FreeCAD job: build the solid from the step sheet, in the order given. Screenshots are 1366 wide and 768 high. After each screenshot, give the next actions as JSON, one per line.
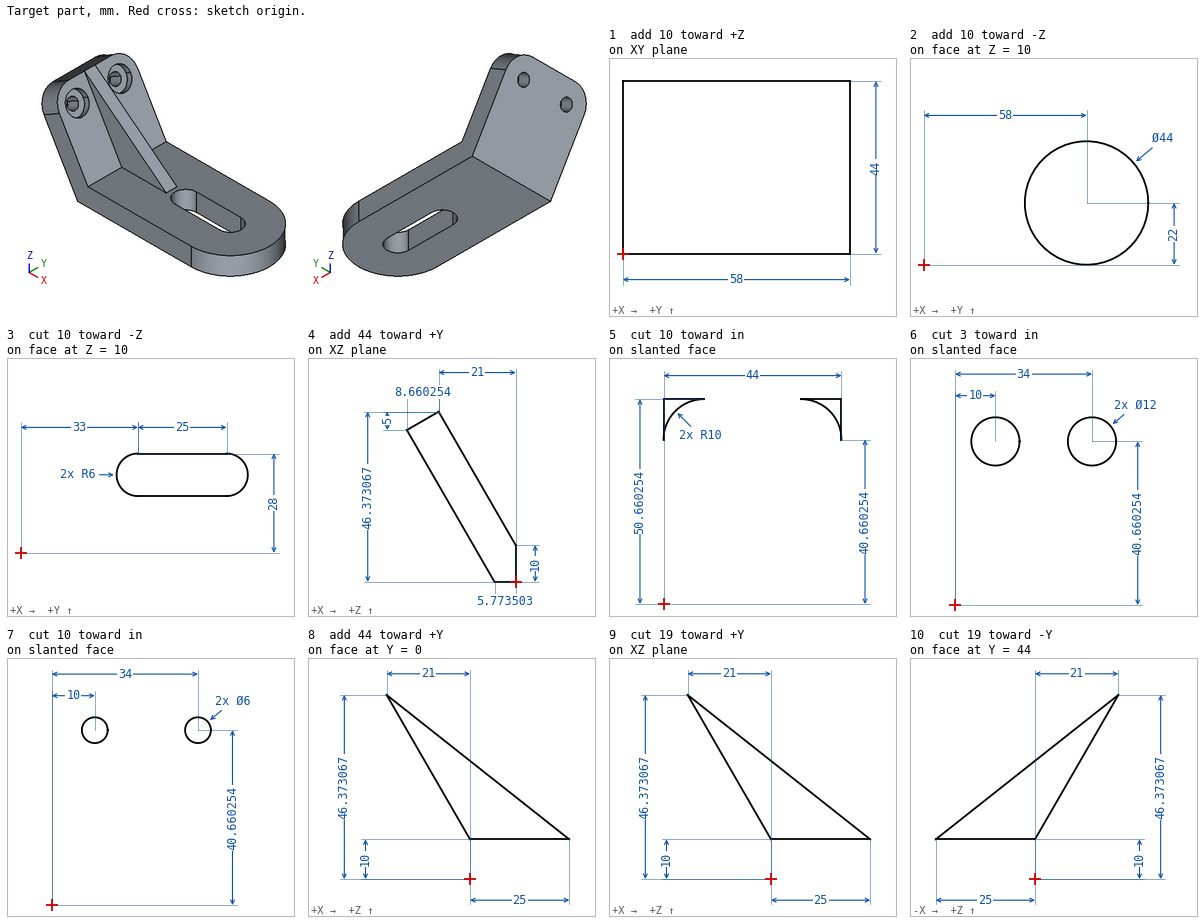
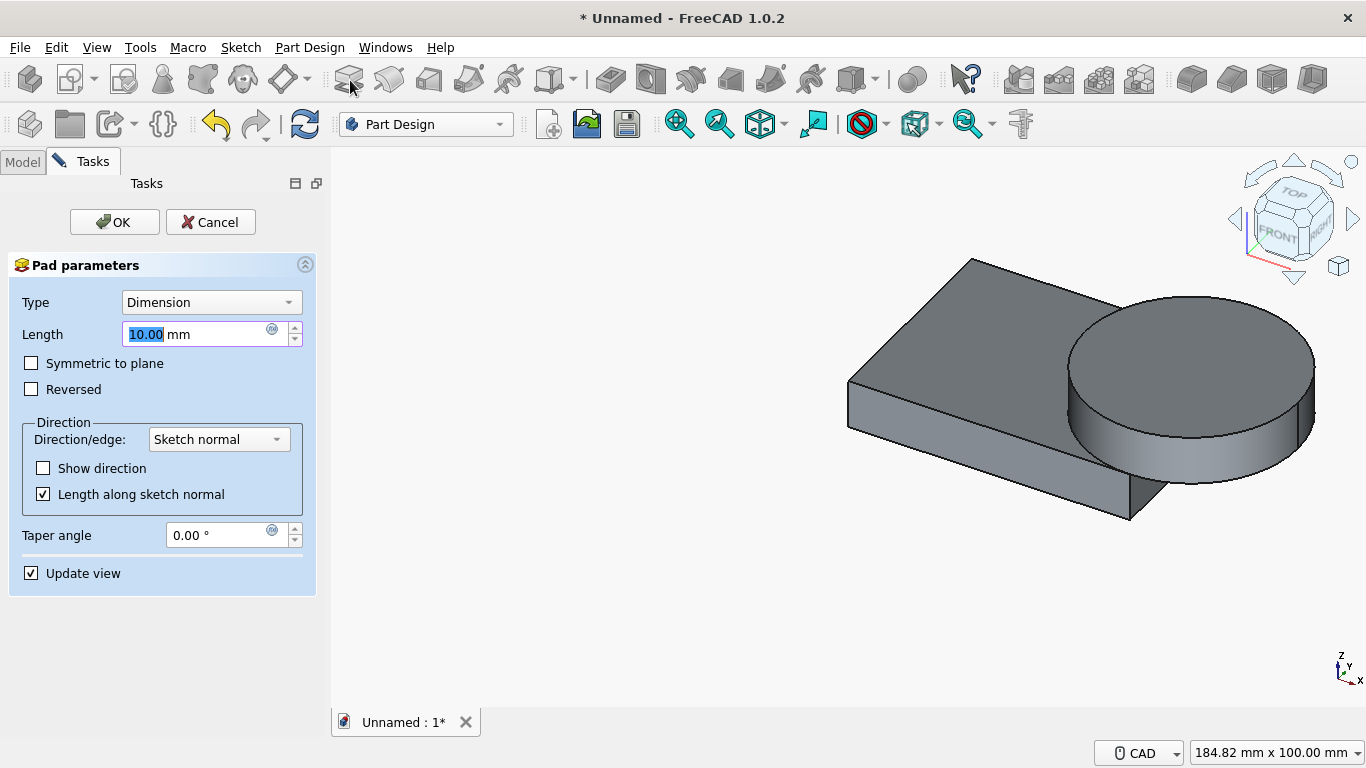
{"action": "type", "text": "10"}
{"action": "key", "text": "Tab"}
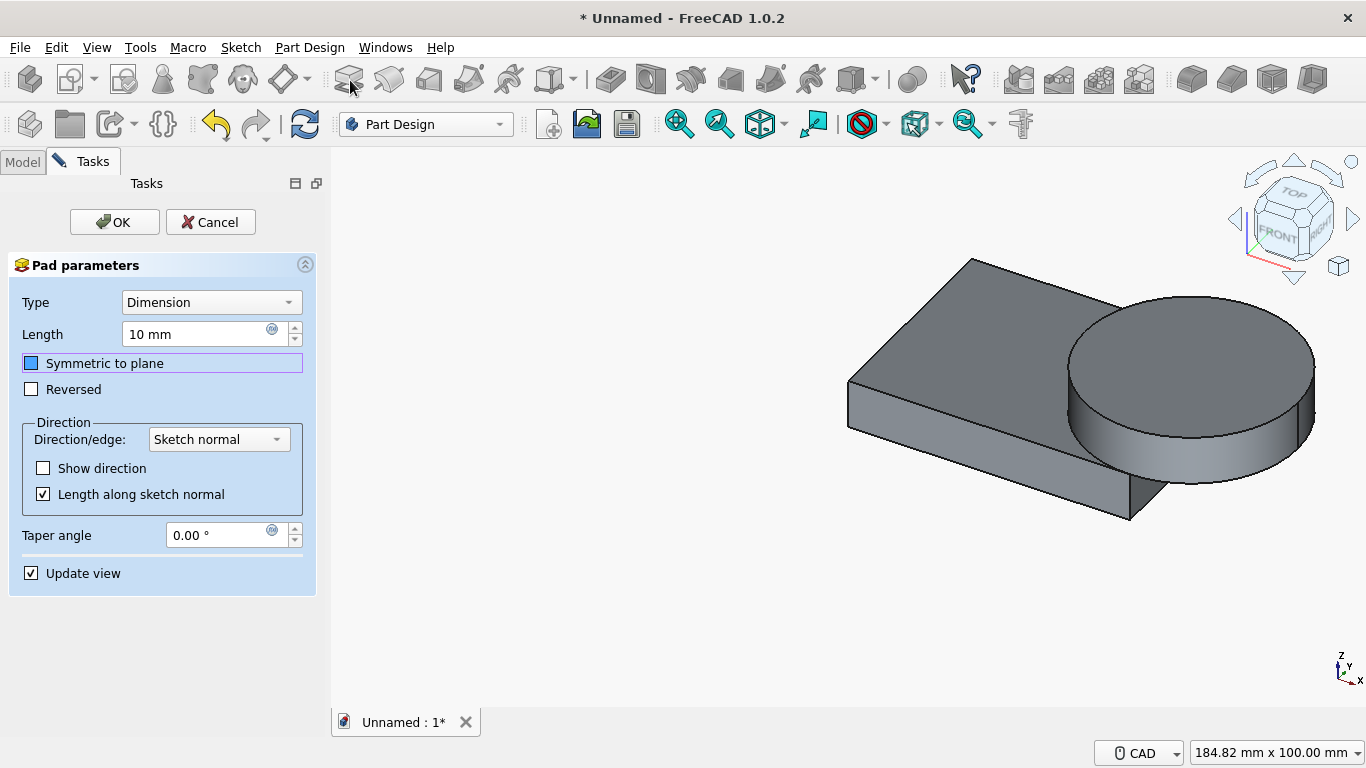
{"action": "left_click", "coordinate": [30, 389]}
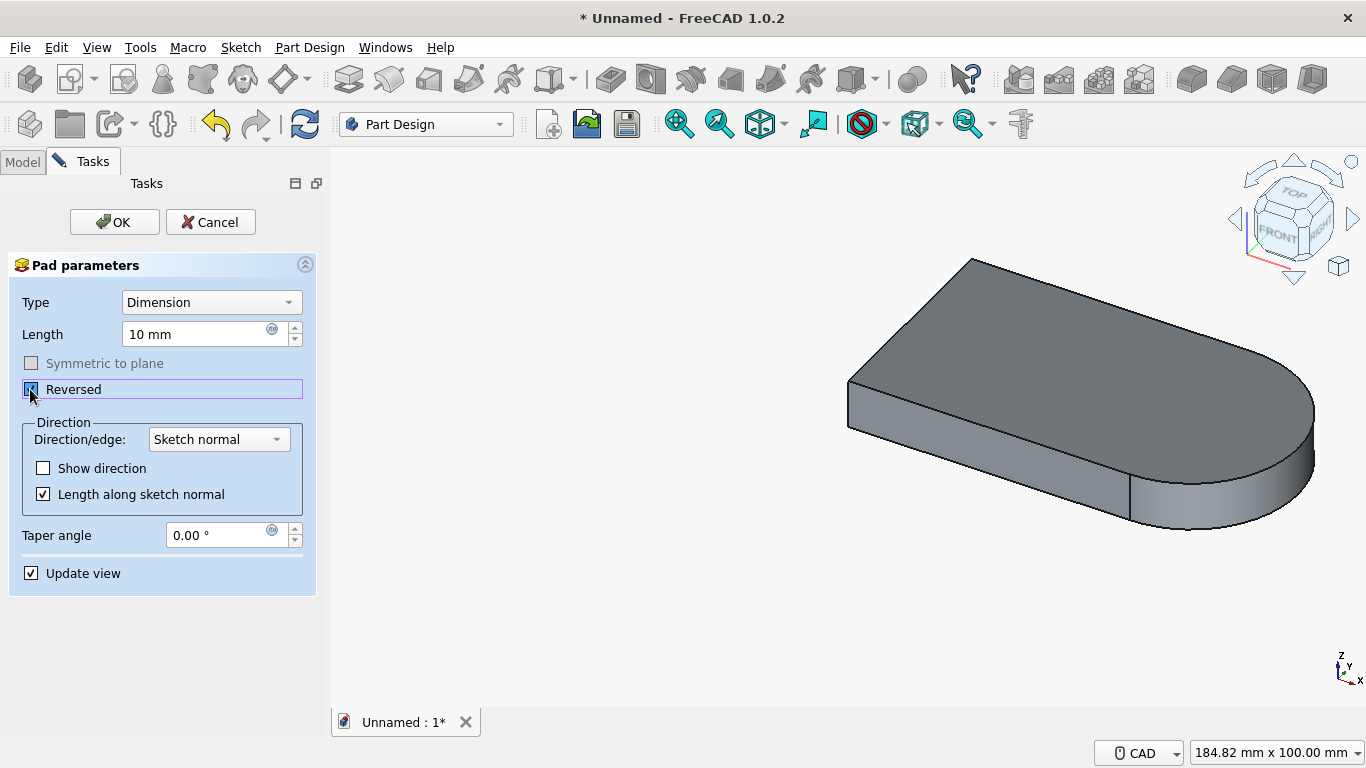
{"action": "left_click", "coordinate": [115, 222]}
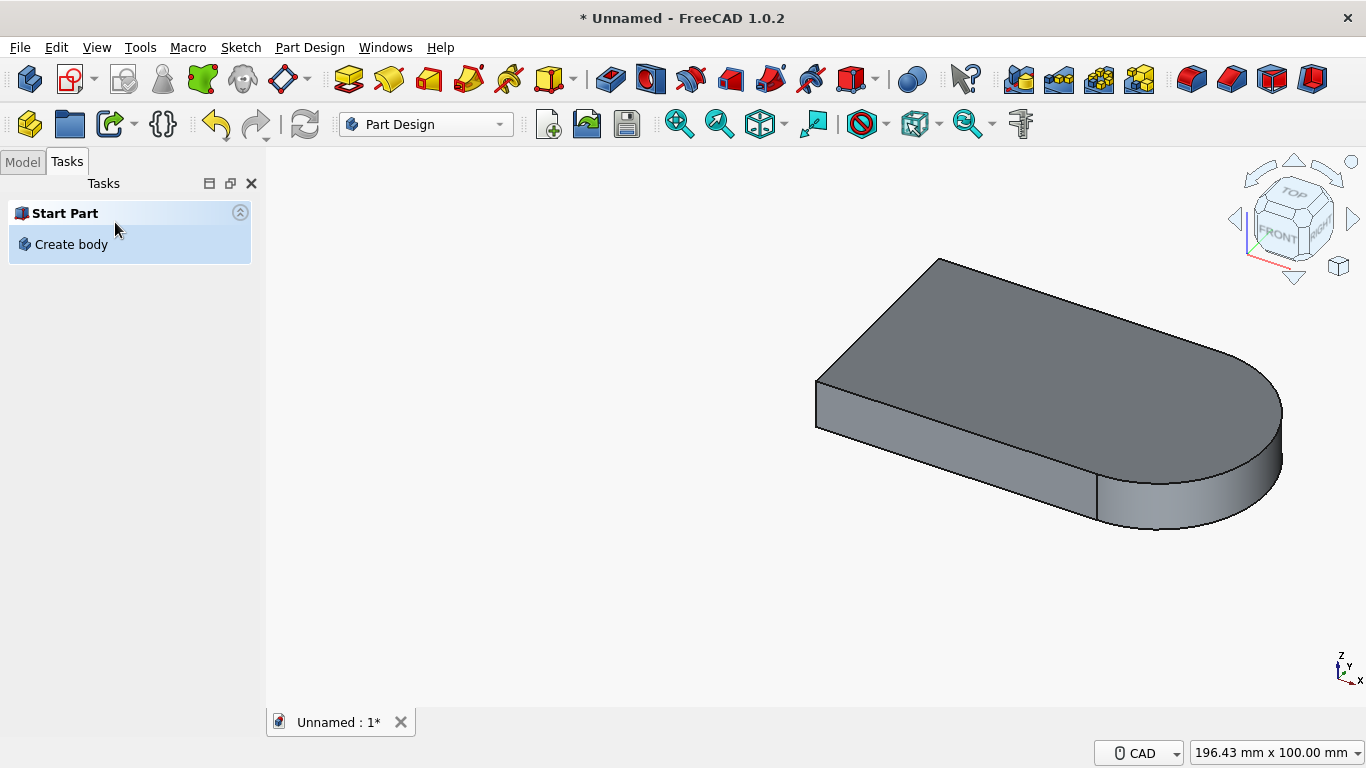
{"action": "left_click", "coordinate": [1127, 402]}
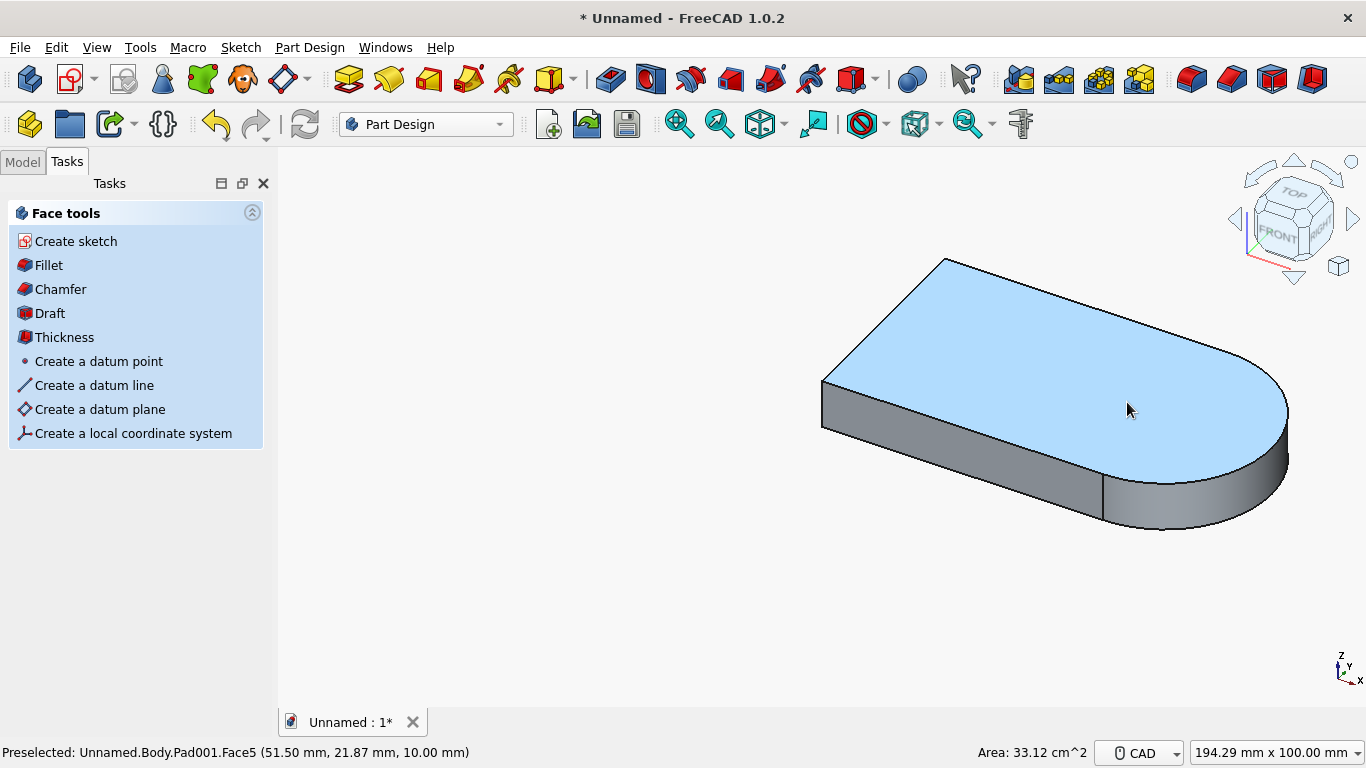
{"action": "left_click", "coordinate": [70, 80]}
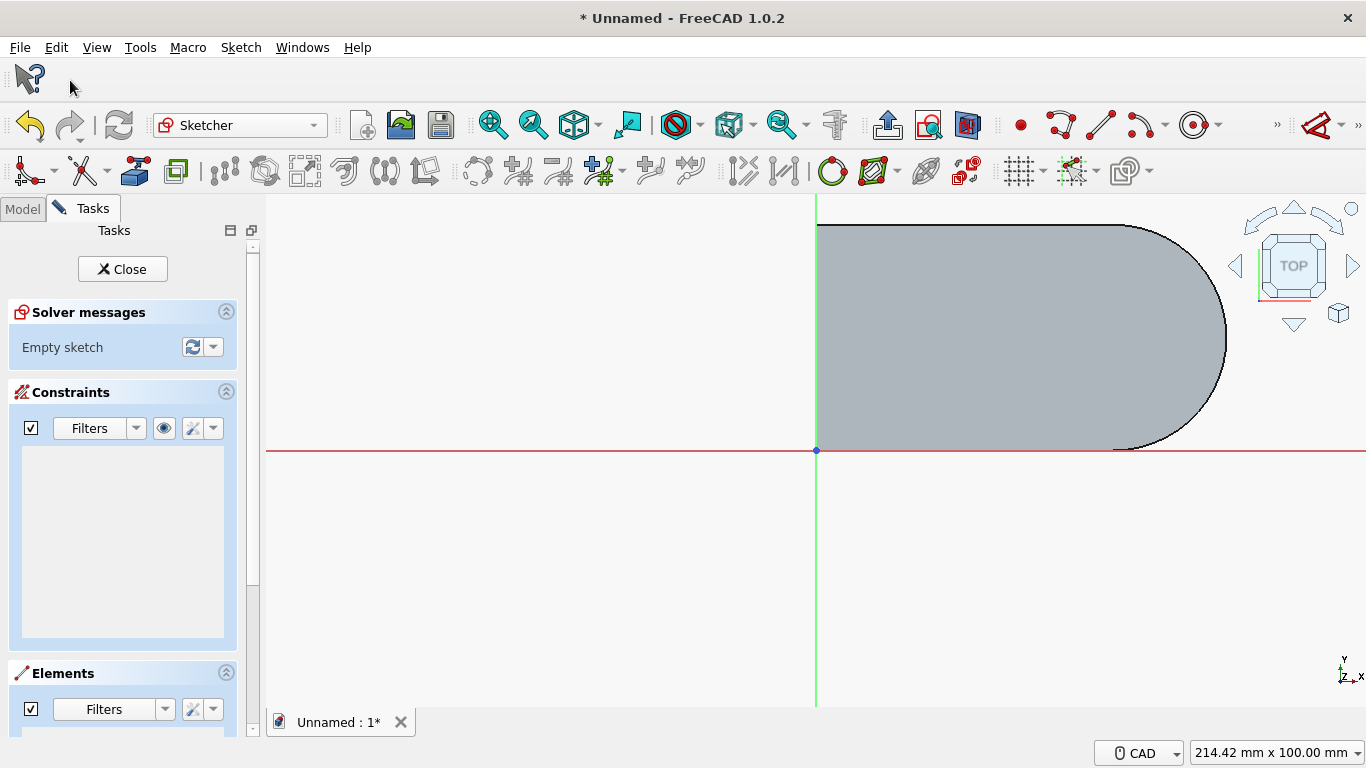
{"action": "scroll", "coordinate": [1201, 291], "scroll_direction": "up", "scroll_amount": 3}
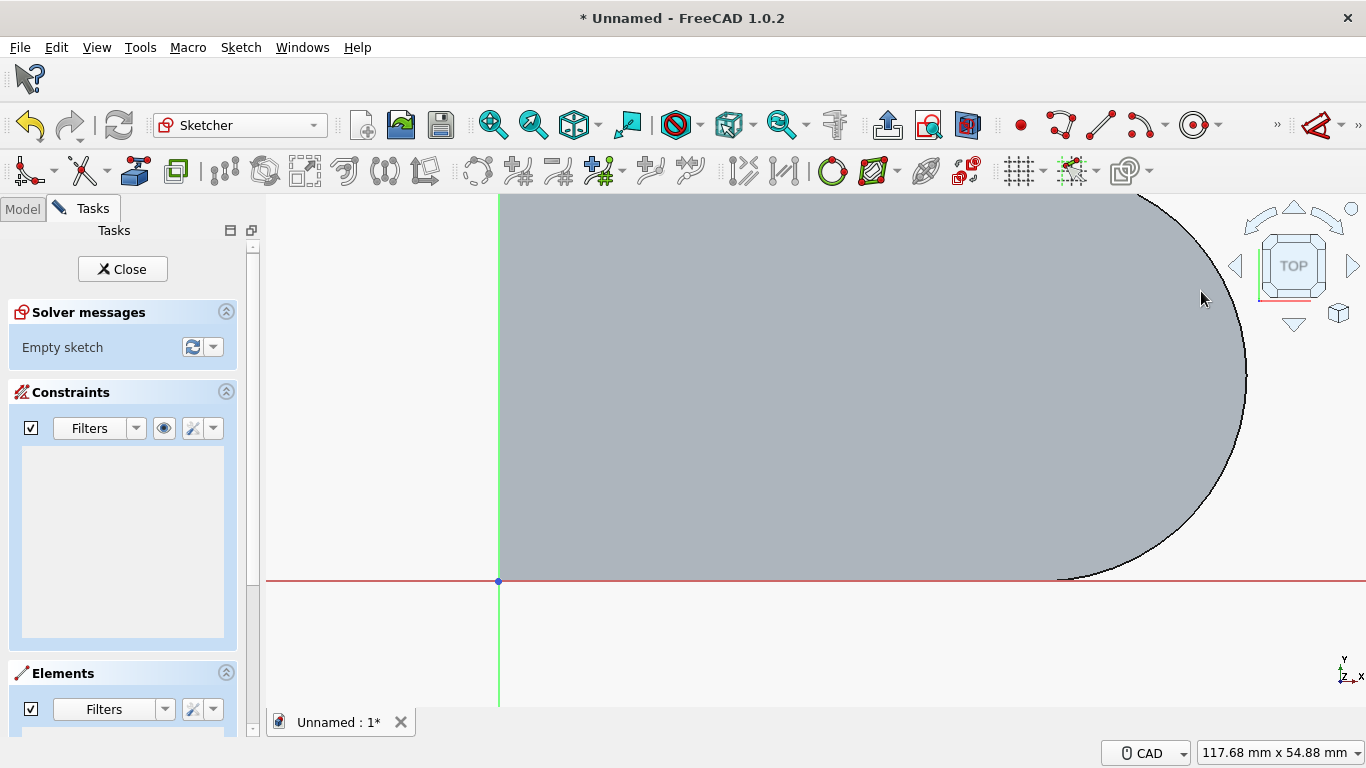
{"action": "key", "text": "g s"}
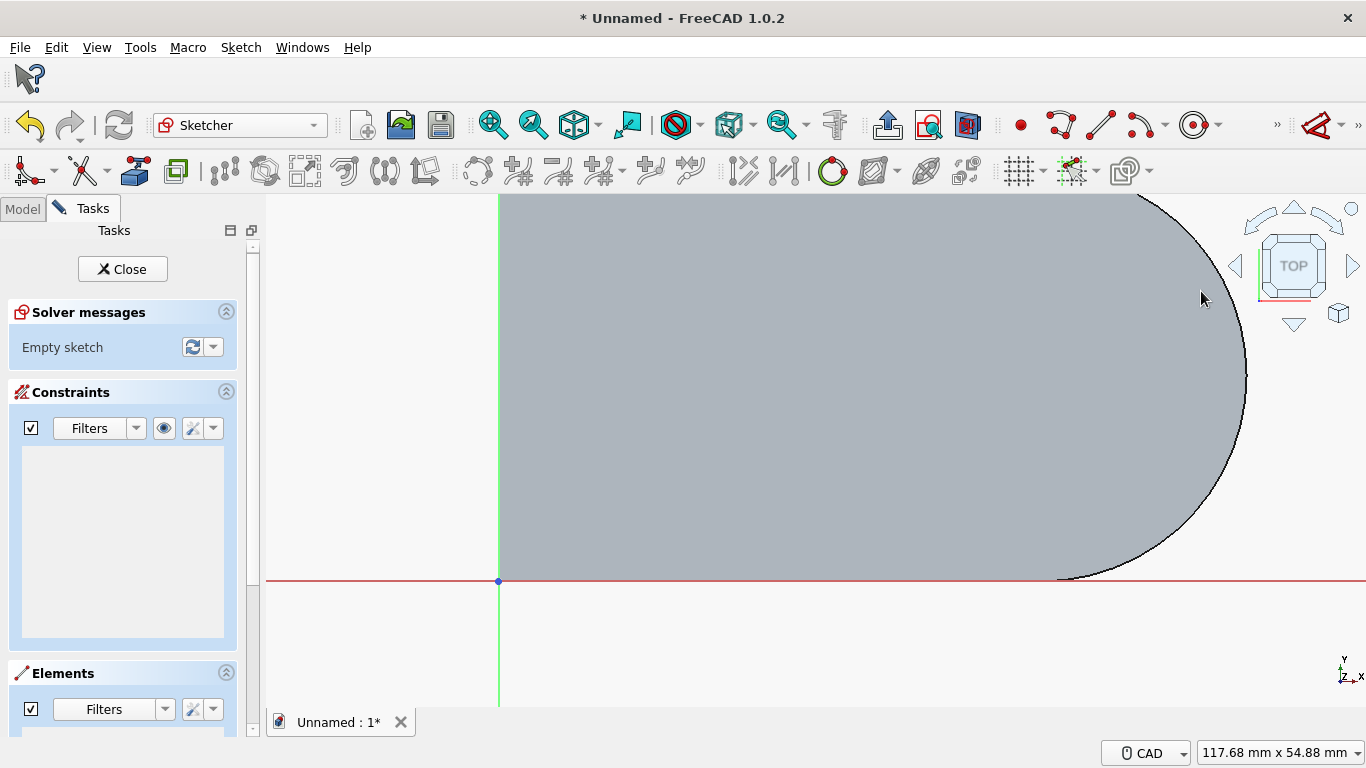
{"action": "left_click", "coordinate": [807, 376]}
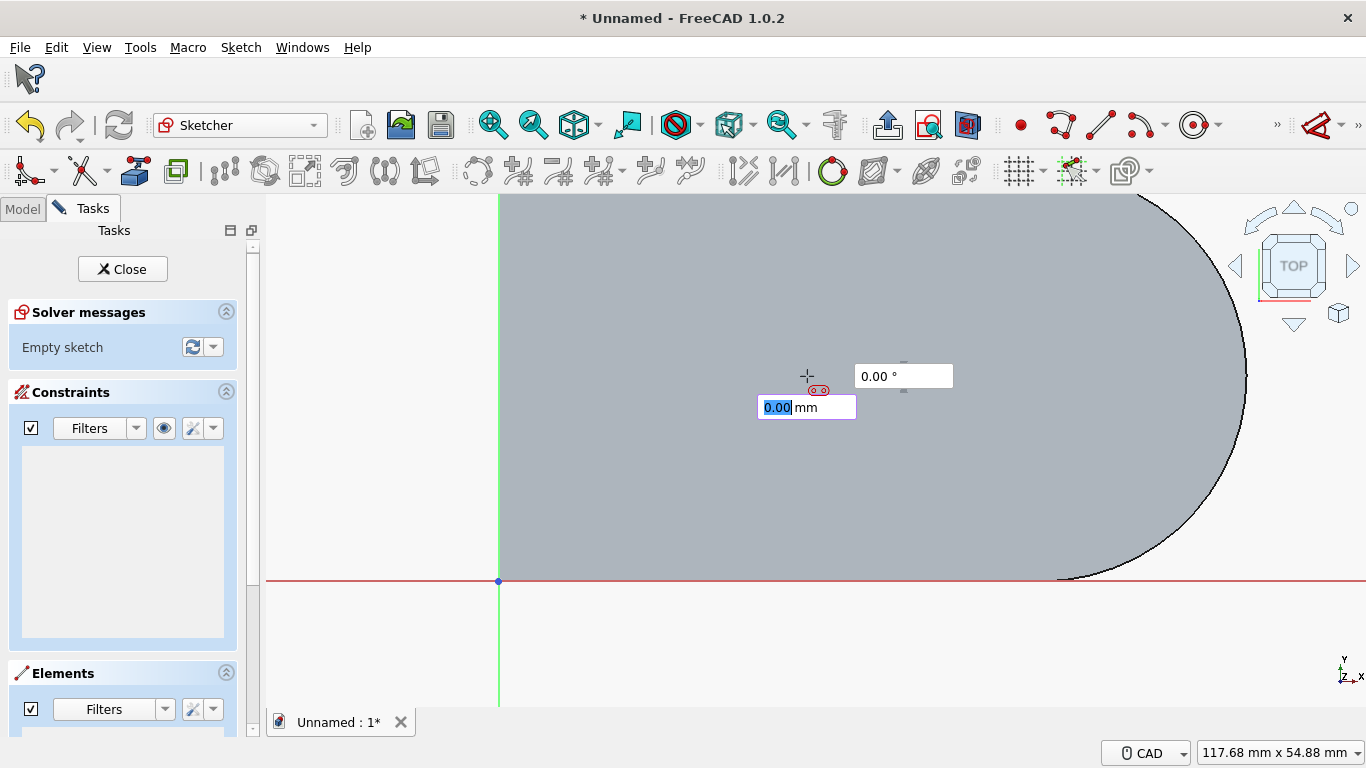
{"action": "left_click", "coordinate": [1041, 376]}